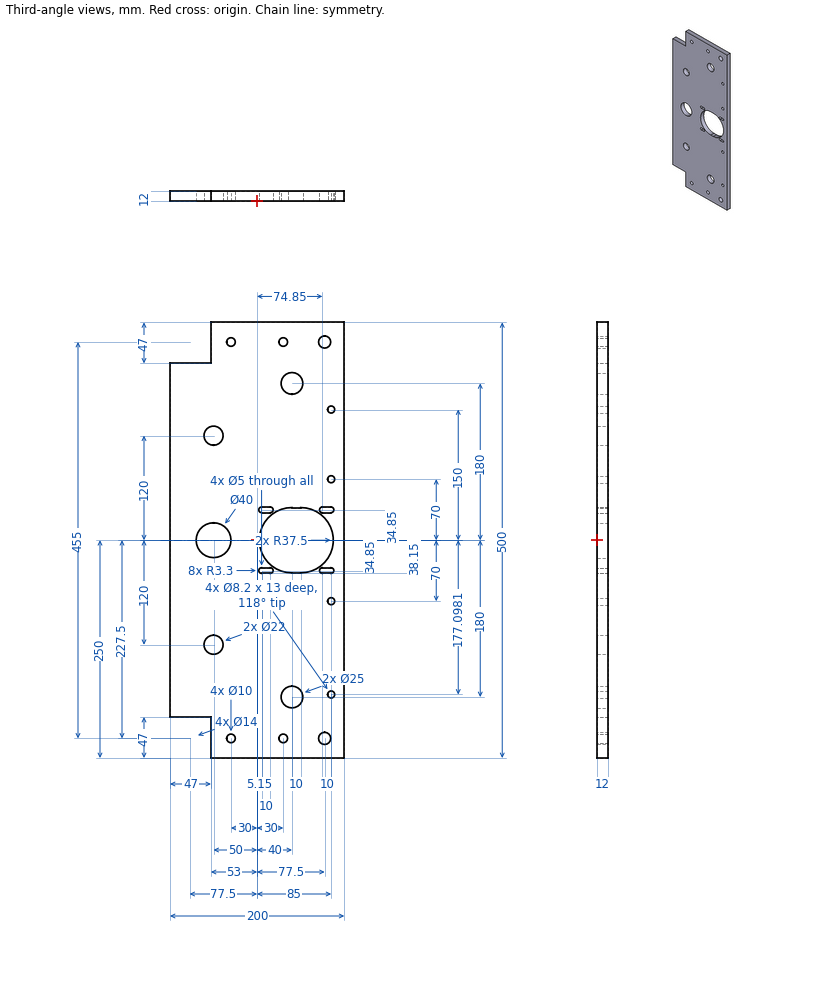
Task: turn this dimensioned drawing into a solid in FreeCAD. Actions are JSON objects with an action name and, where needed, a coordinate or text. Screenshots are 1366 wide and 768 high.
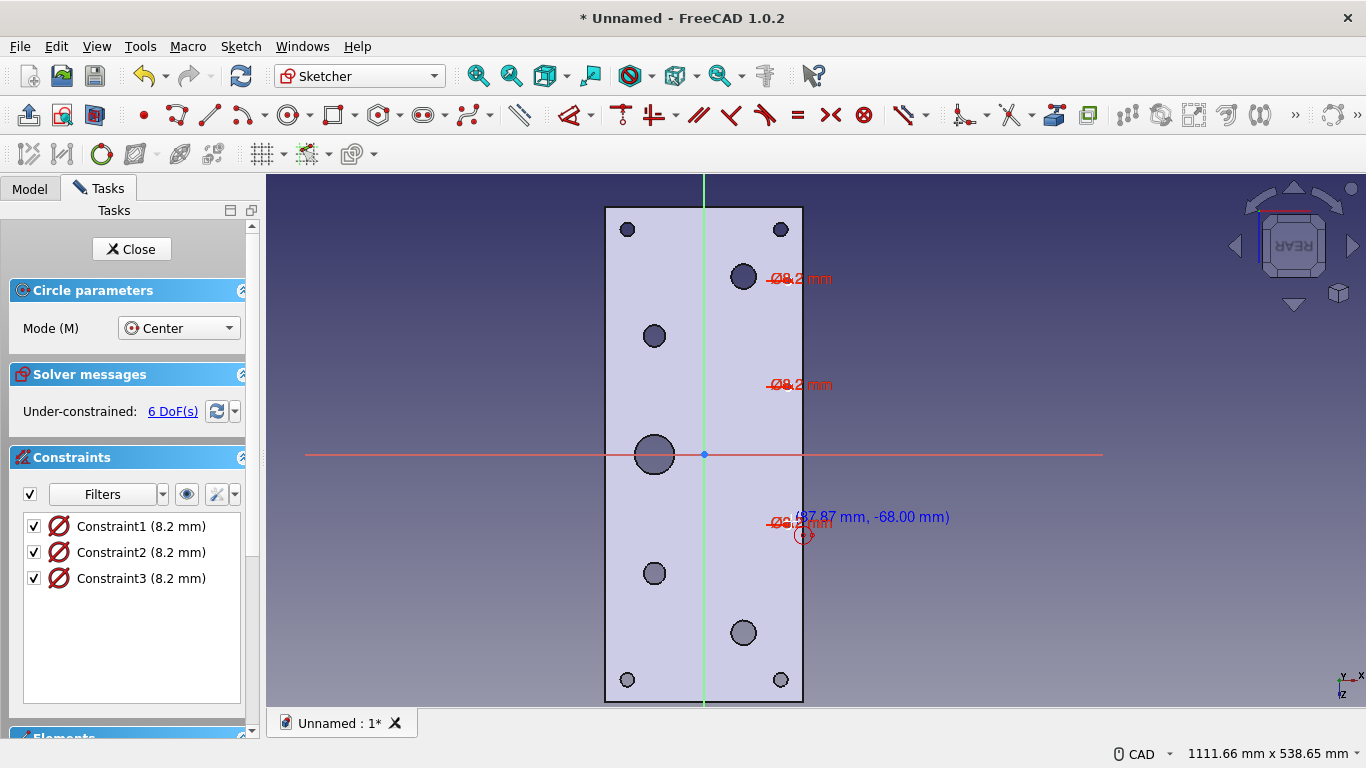
{"action": "scroll", "coordinate": [788, 603], "scroll_direction": "up", "scroll_amount": 9}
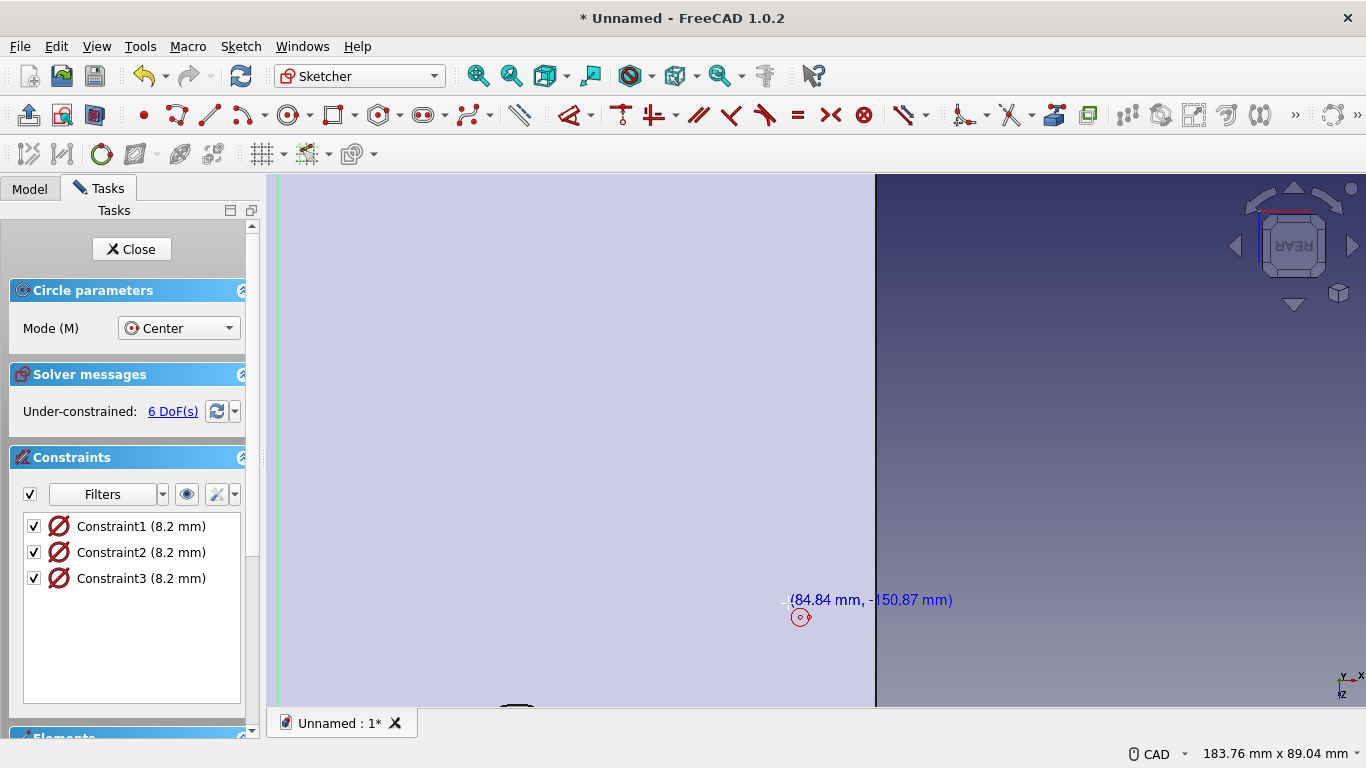
{"action": "scroll", "coordinate": [788, 603], "scroll_direction": "down", "scroll_amount": 9}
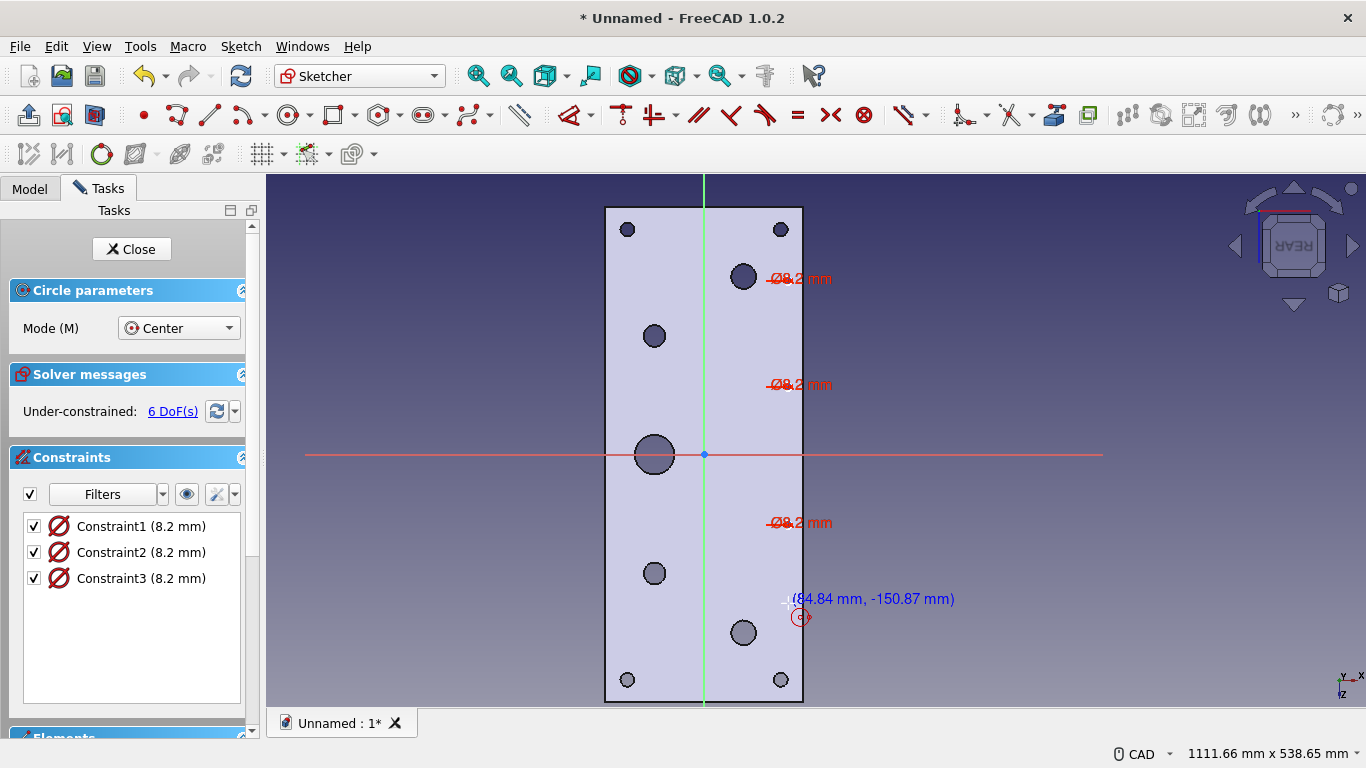
{"action": "left_click", "coordinate": [788, 603]}
{"action": "mouse_move", "coordinate": [791, 600]}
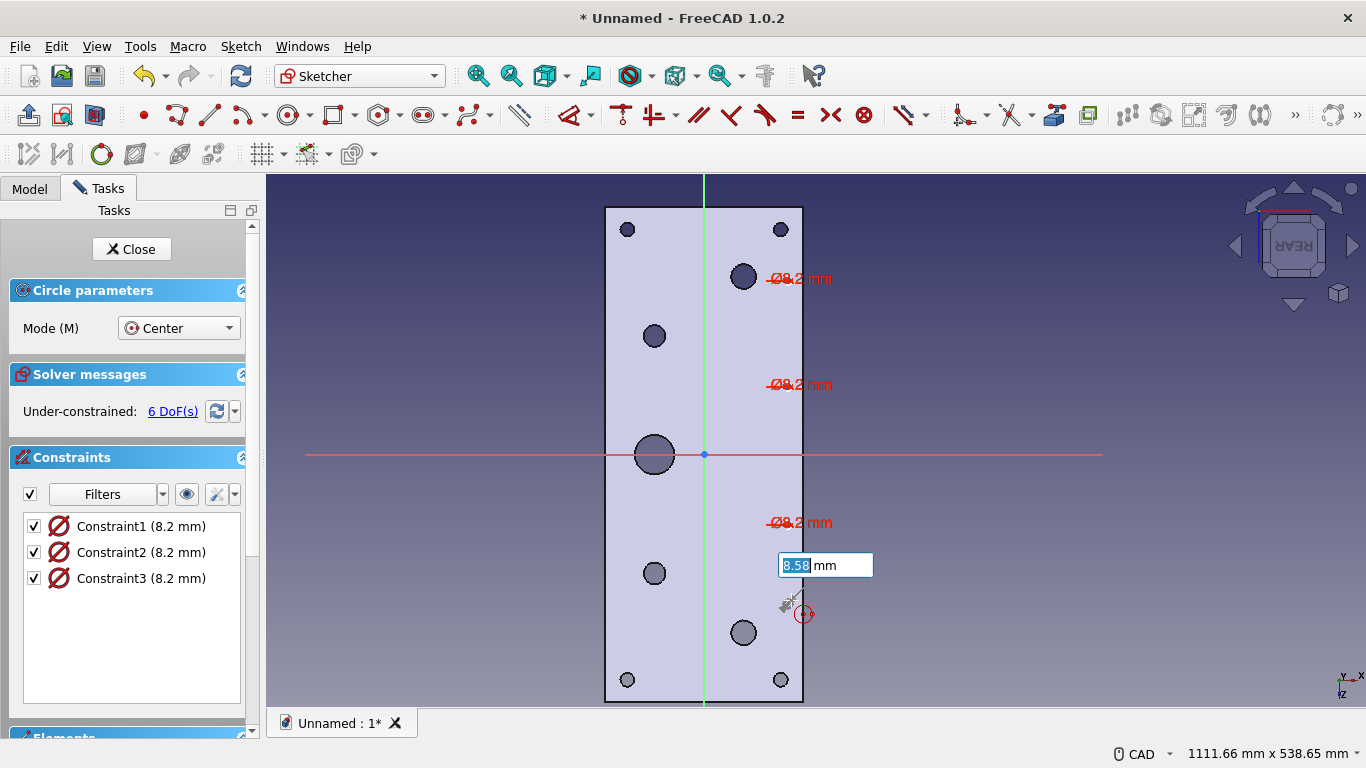
{"action": "type", "text": "8.2"}
{"action": "key", "text": "Return"}
{"action": "key", "text": "Escape"}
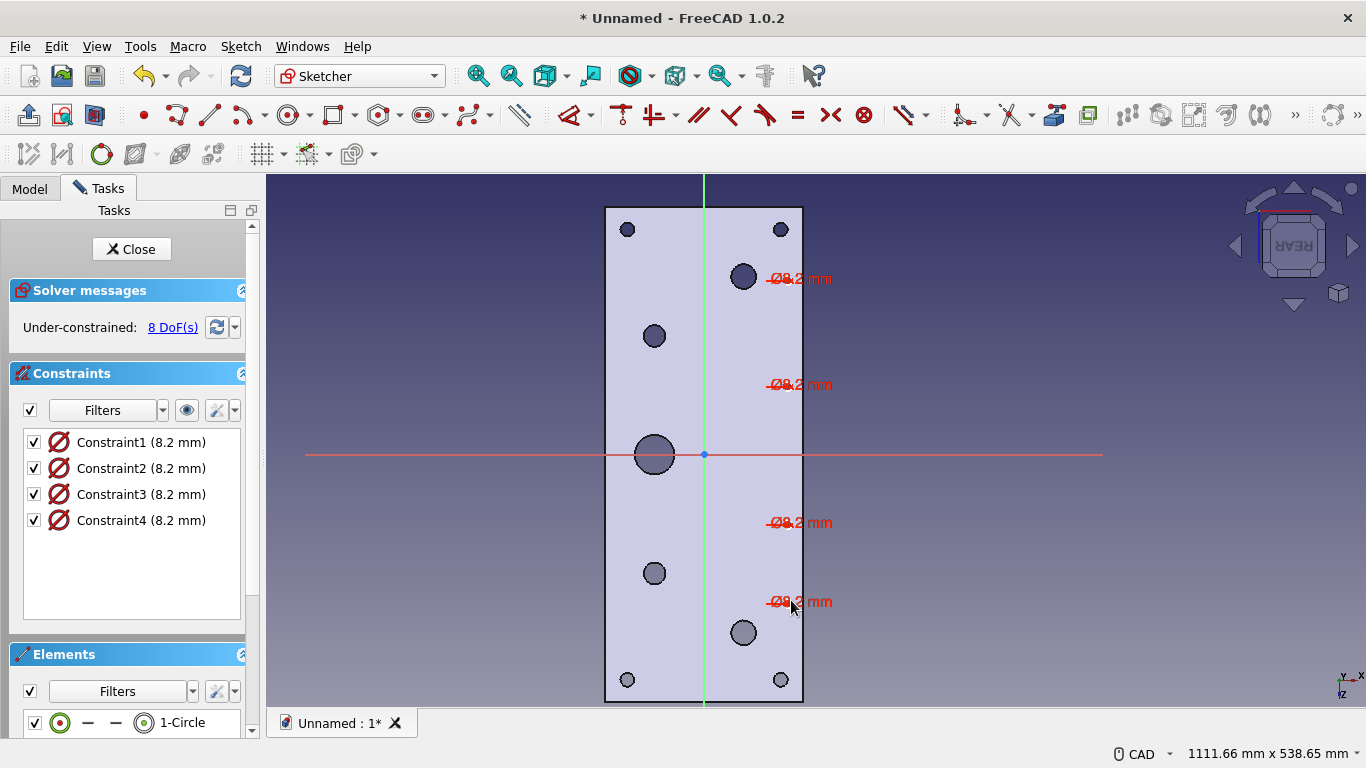
{"action": "left_click", "coordinate": [788, 281]}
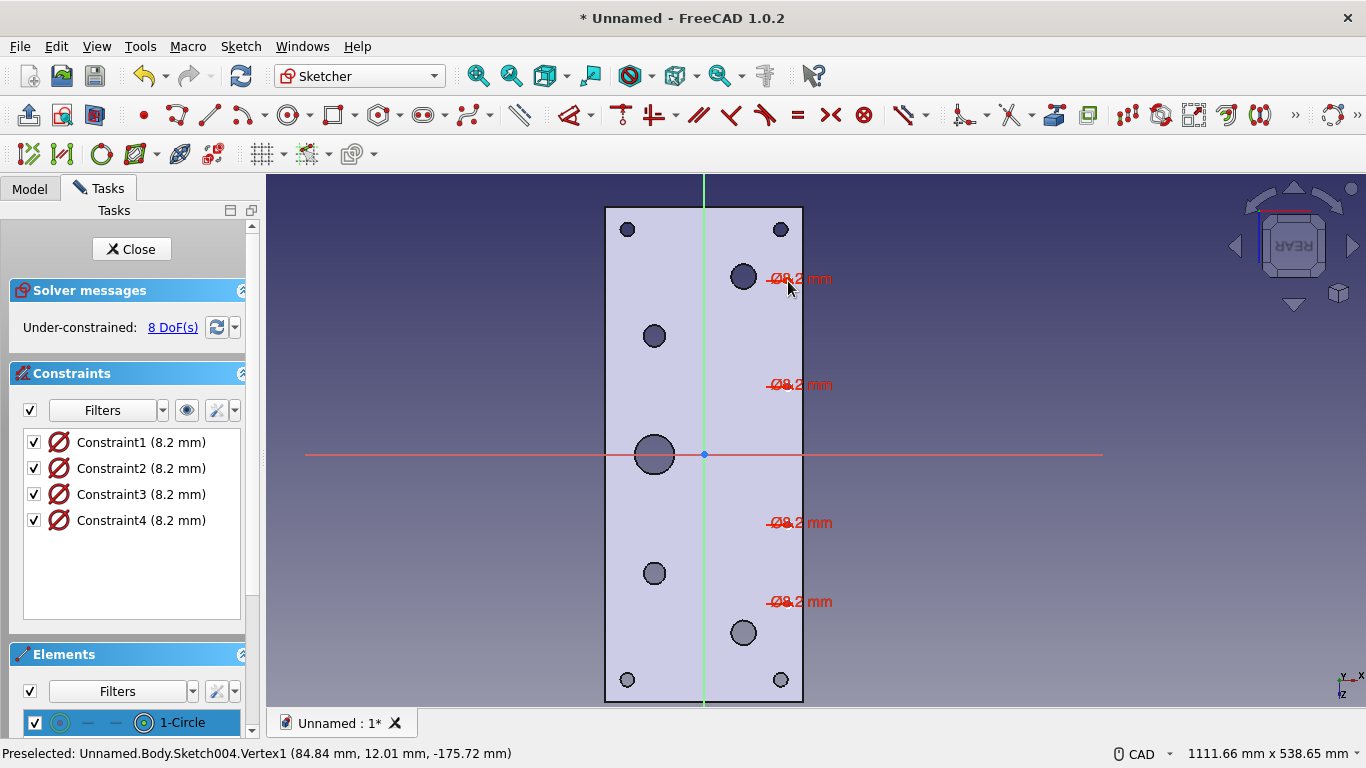
{"action": "left_click", "coordinate": [788, 387]}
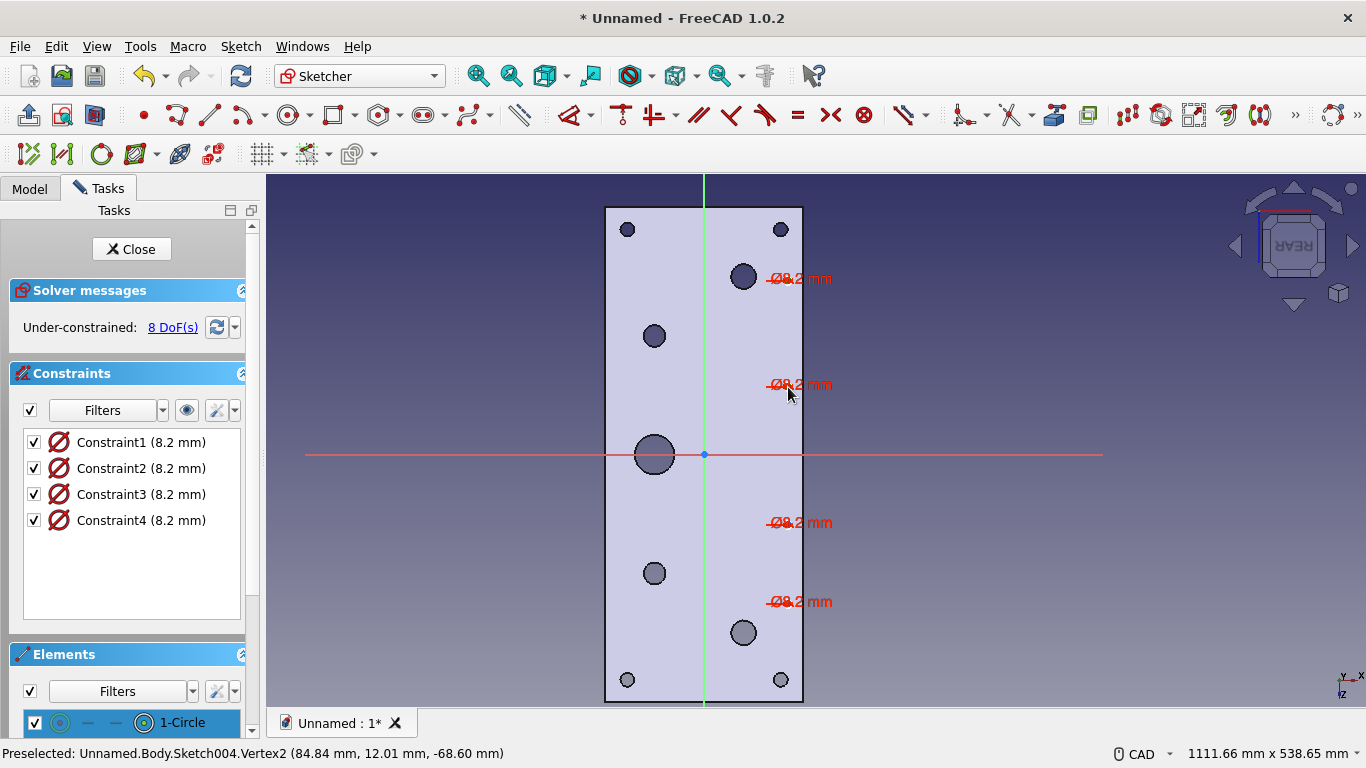
{"action": "left_click", "coordinate": [676, 116]}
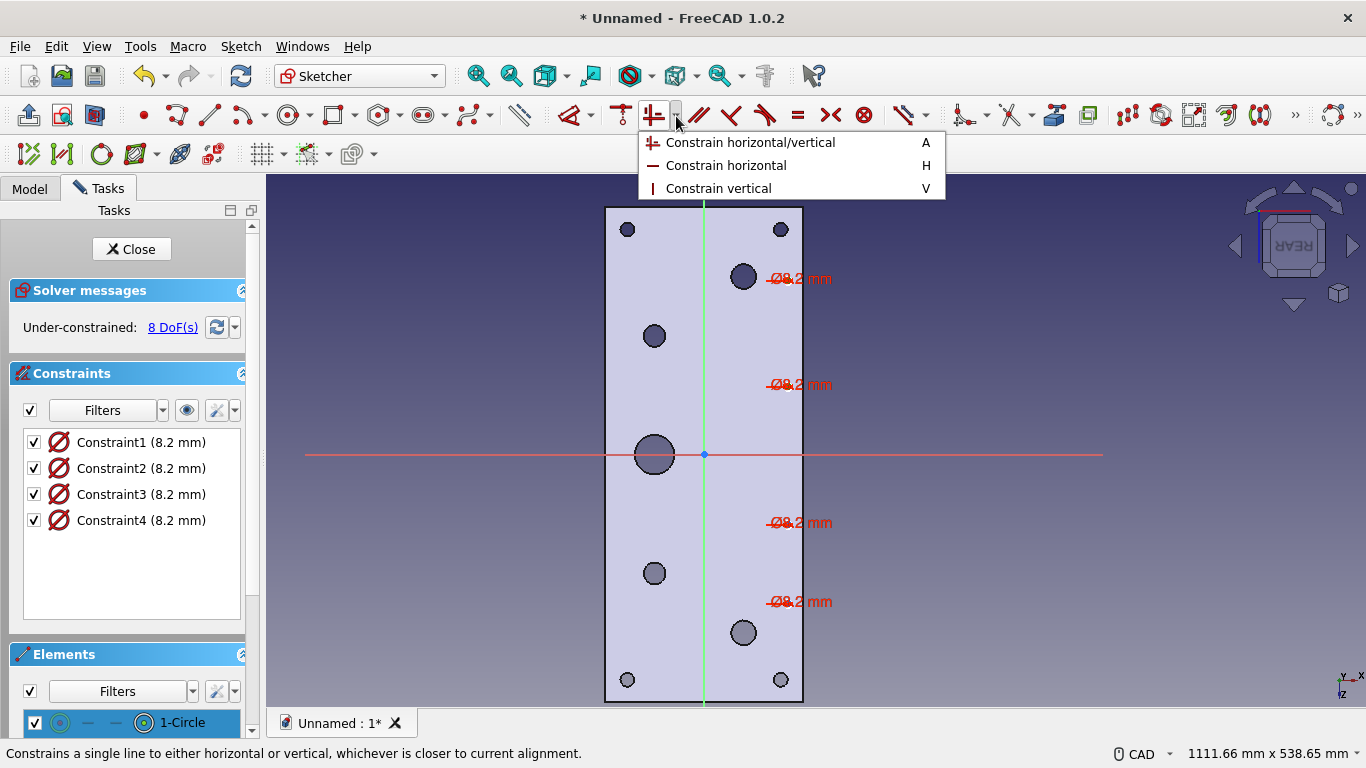
{"action": "left_click", "coordinate": [792, 188]}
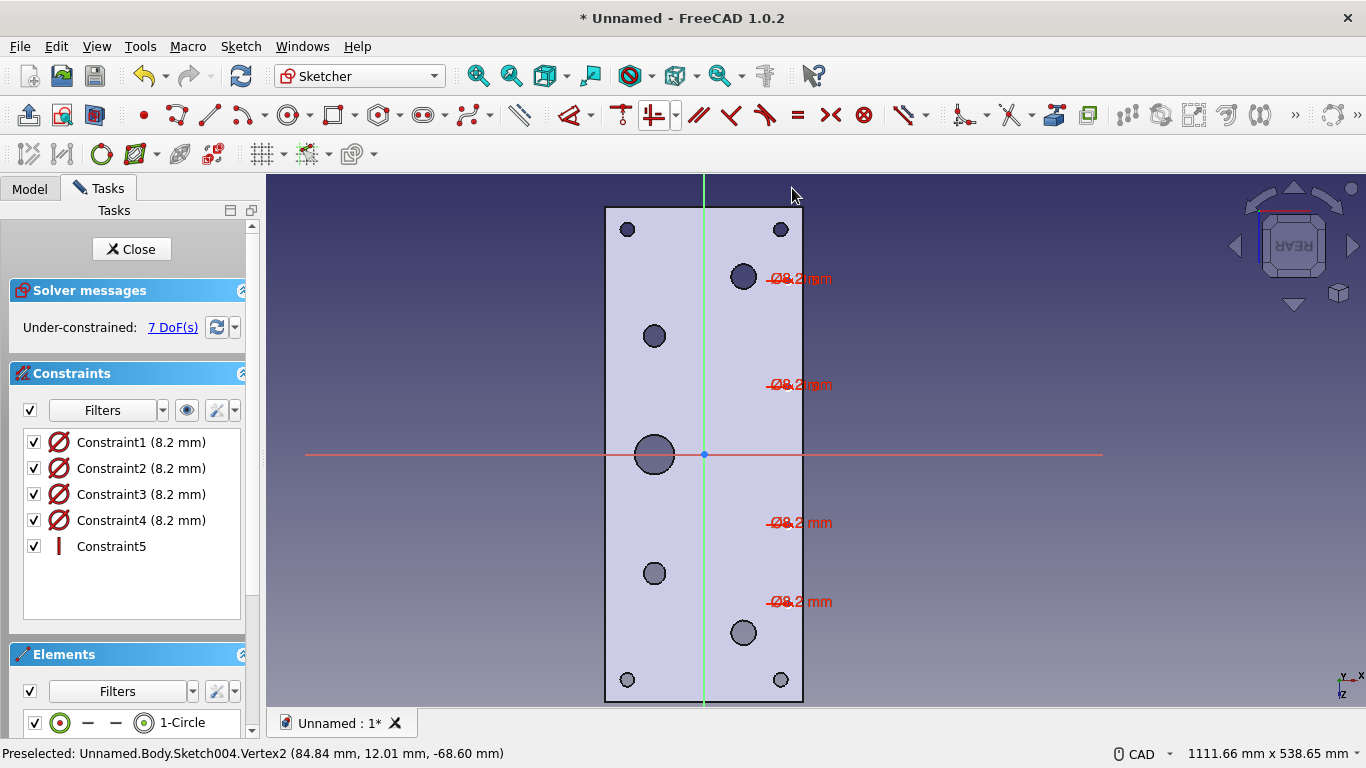
{"action": "left_click", "coordinate": [788, 387]}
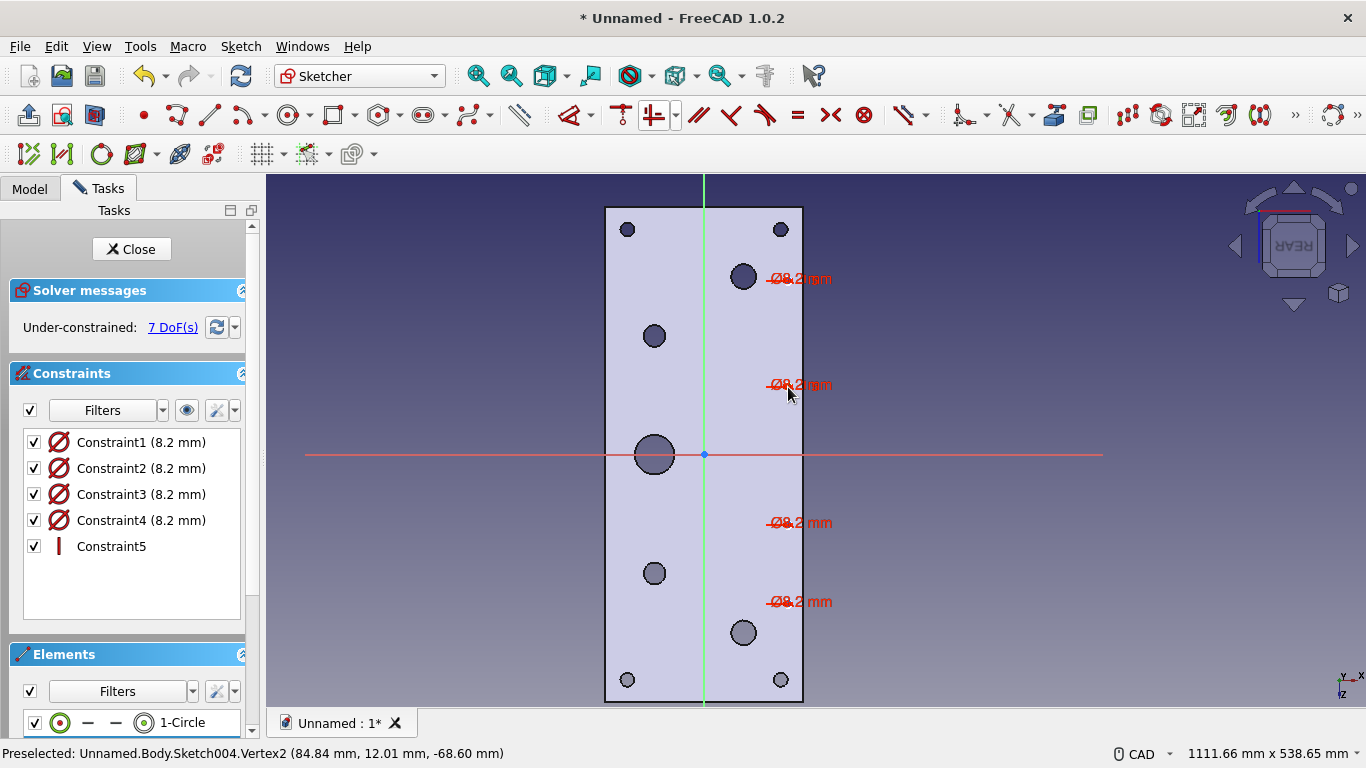
{"action": "left_click", "coordinate": [788, 525]}